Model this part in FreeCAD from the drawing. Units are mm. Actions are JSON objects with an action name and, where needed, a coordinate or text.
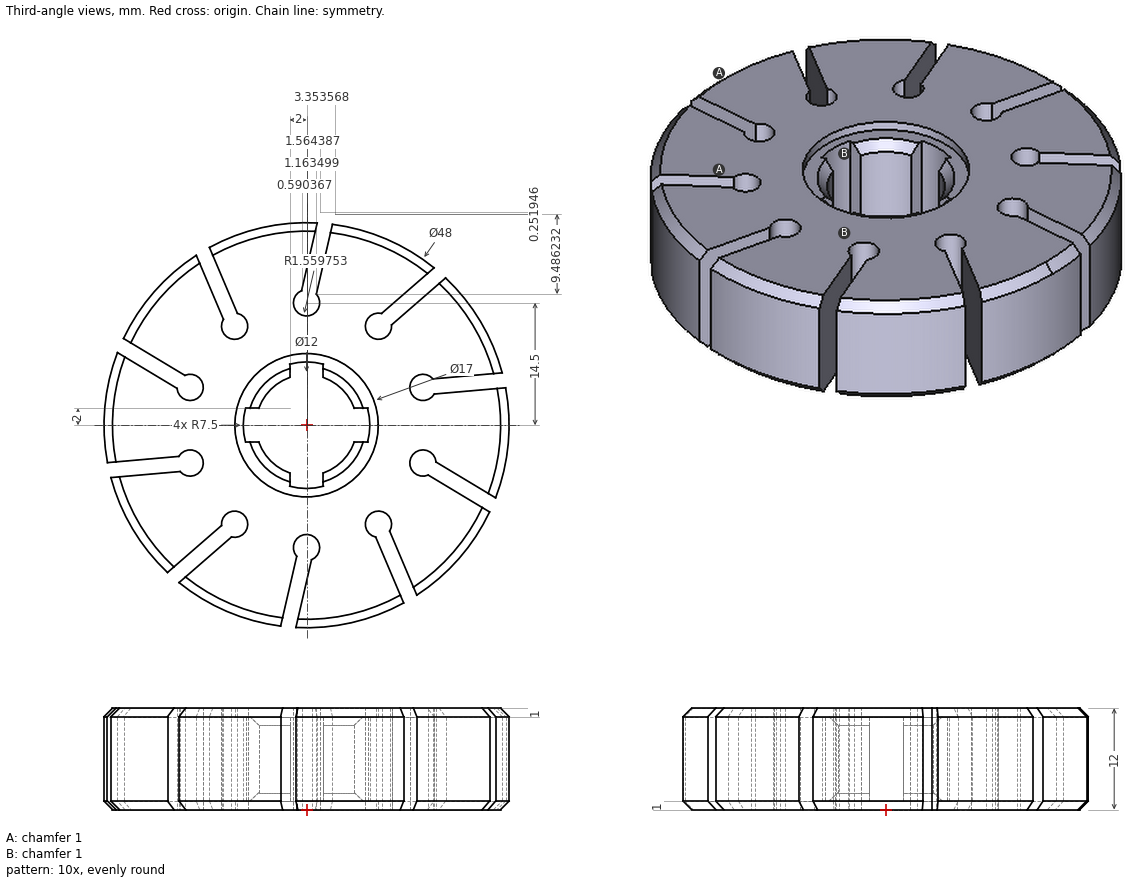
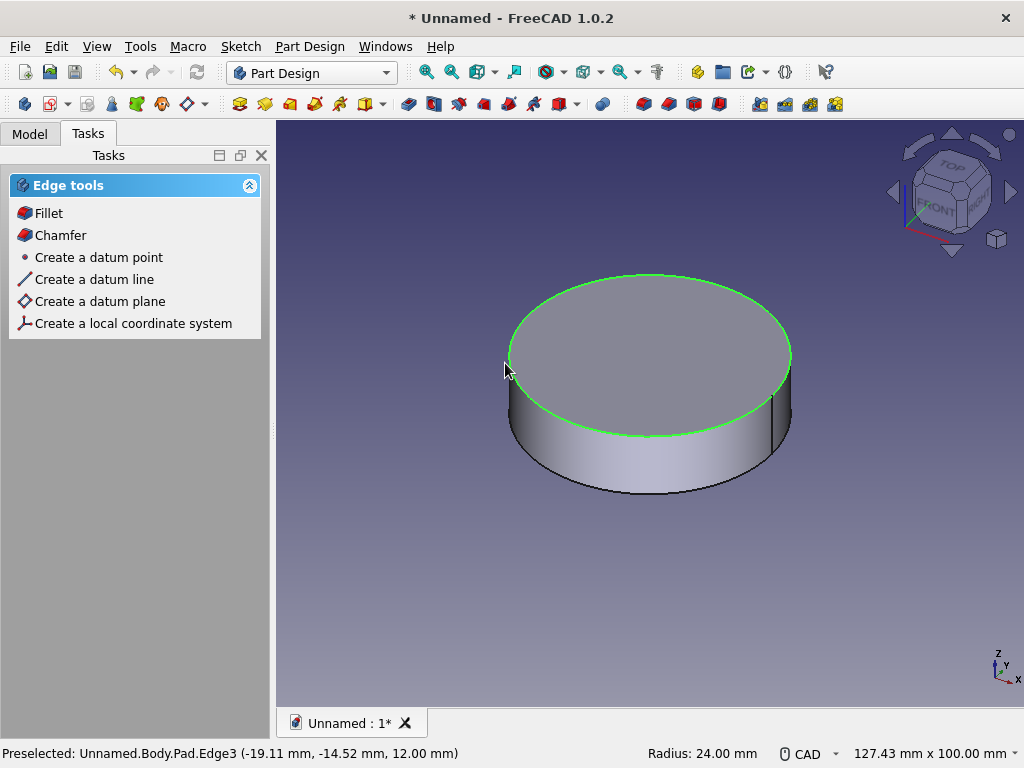
{"action": "key", "text": "0"}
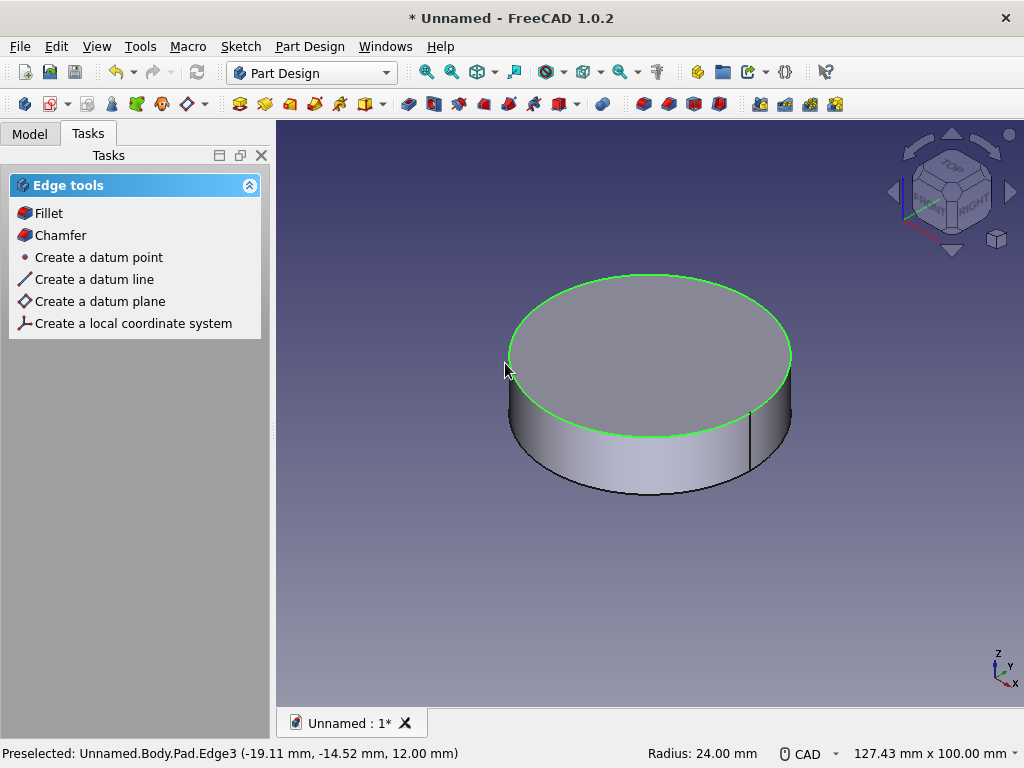
{"action": "key", "text": "2"}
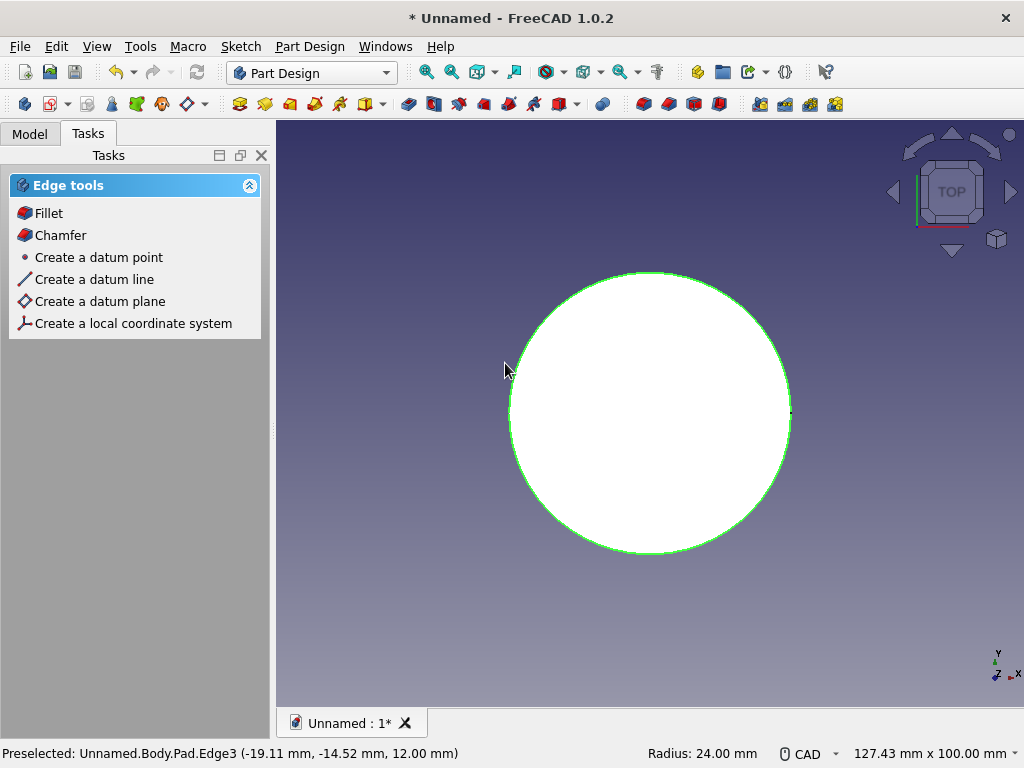
{"action": "key", "text": "1"}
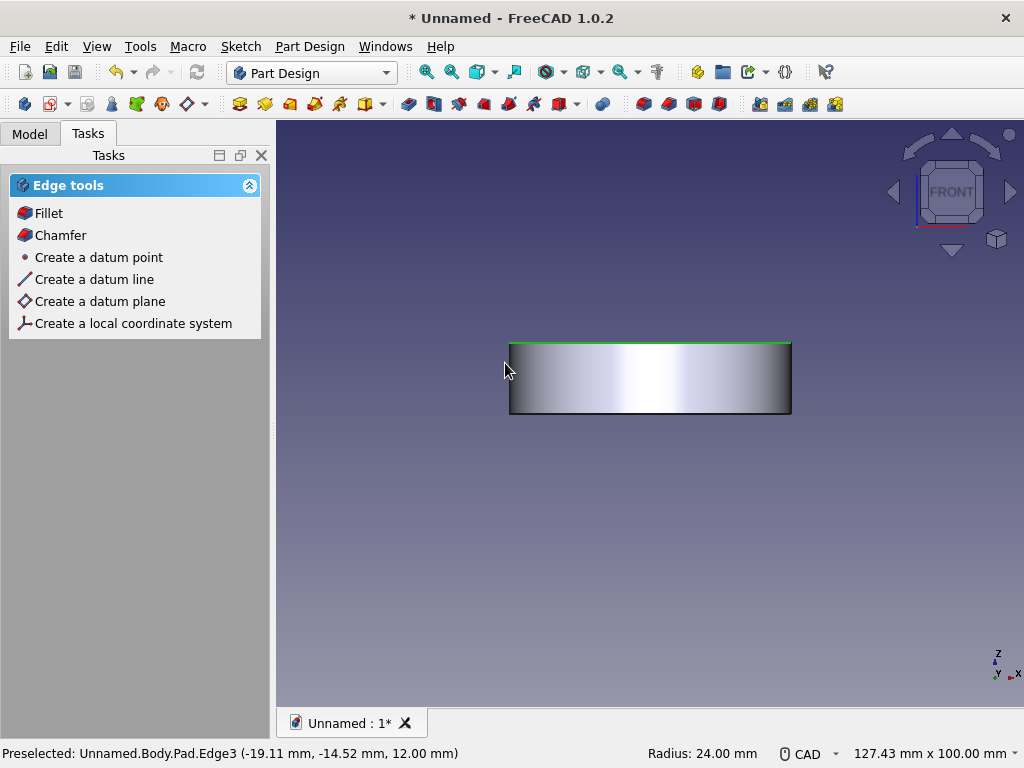
{"action": "left_click", "coordinate": [427, 72]}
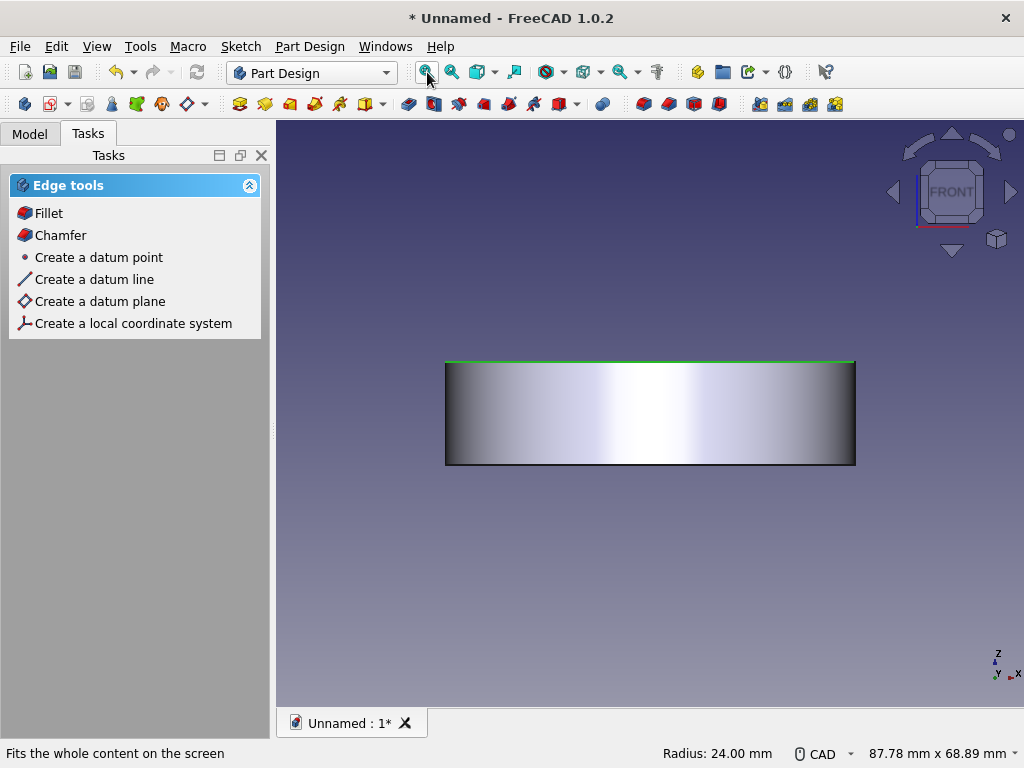
{"action": "left_click", "coordinate": [485, 464], "text": "ctrl"}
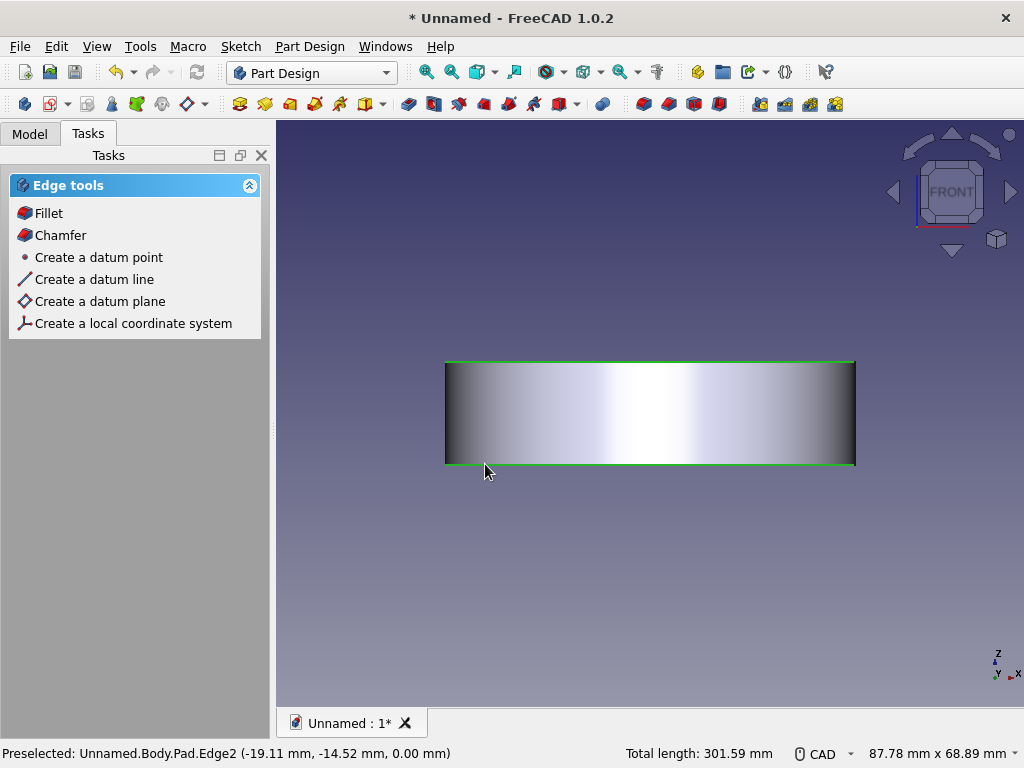
{"action": "left_click", "coordinate": [669, 104]}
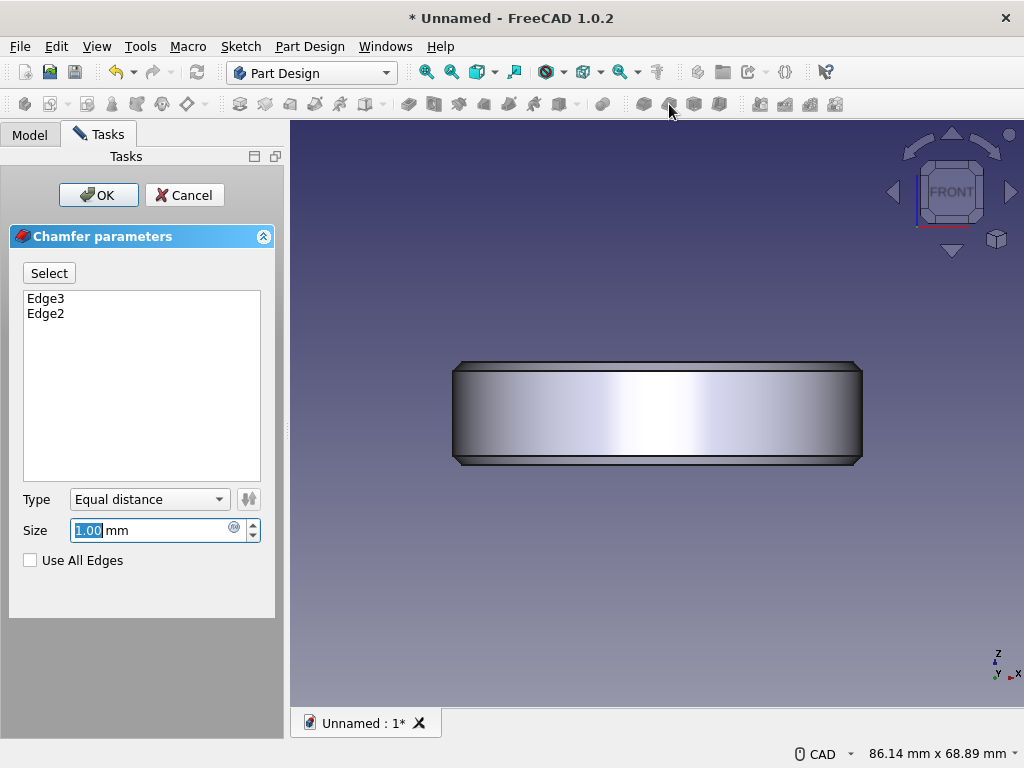
{"action": "type", "text": "1"}
{"action": "key", "text": "Tab"}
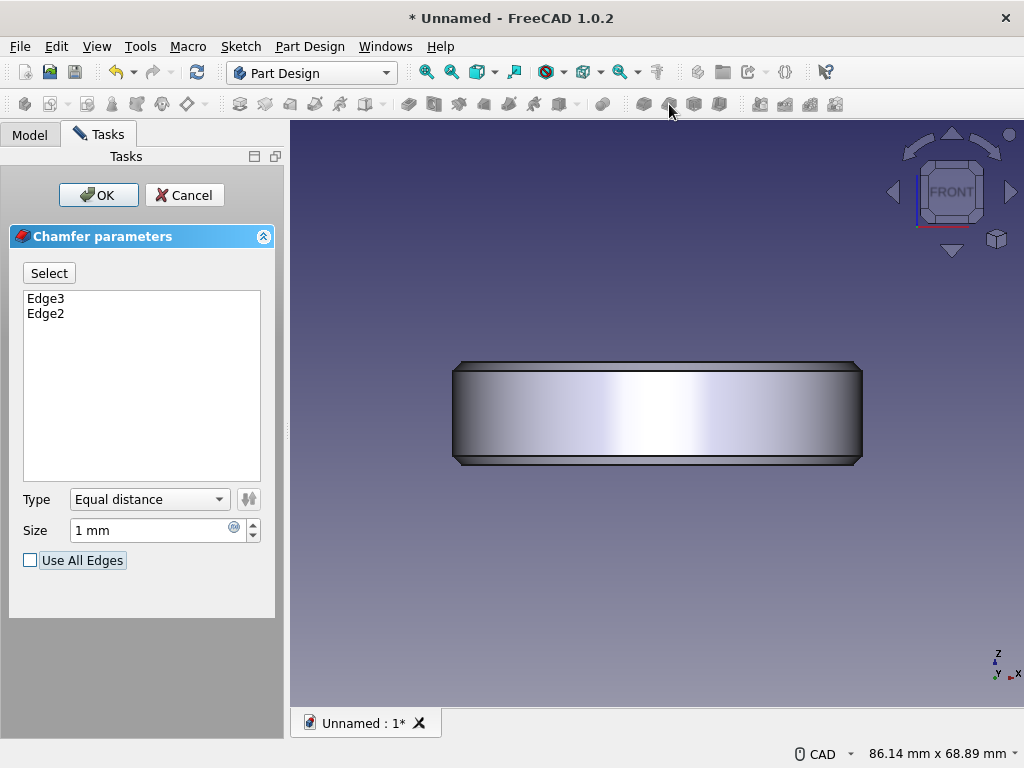
{"action": "left_click", "coordinate": [99, 195]}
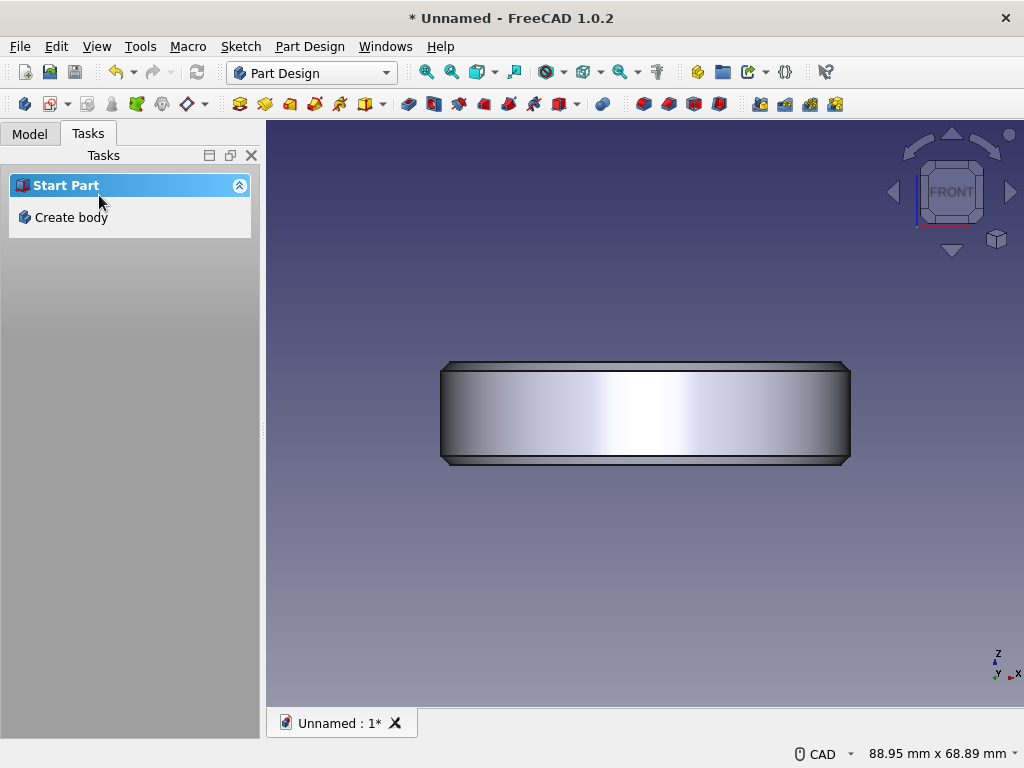
{"action": "key", "text": "0"}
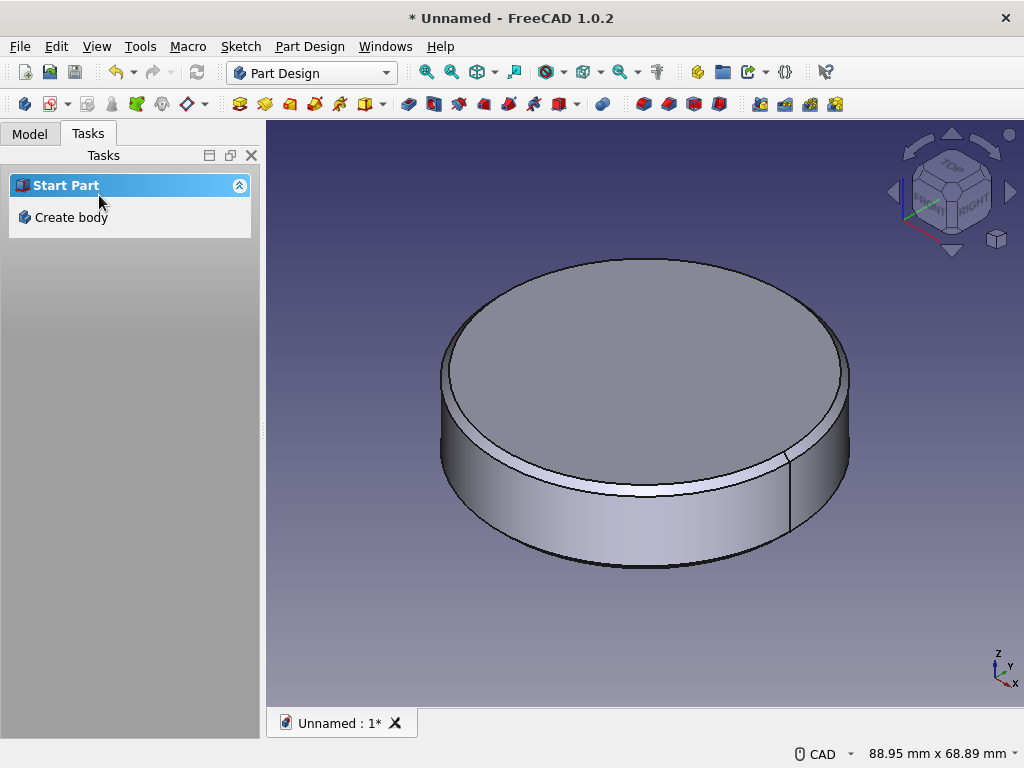
{"action": "left_click", "coordinate": [645, 371]}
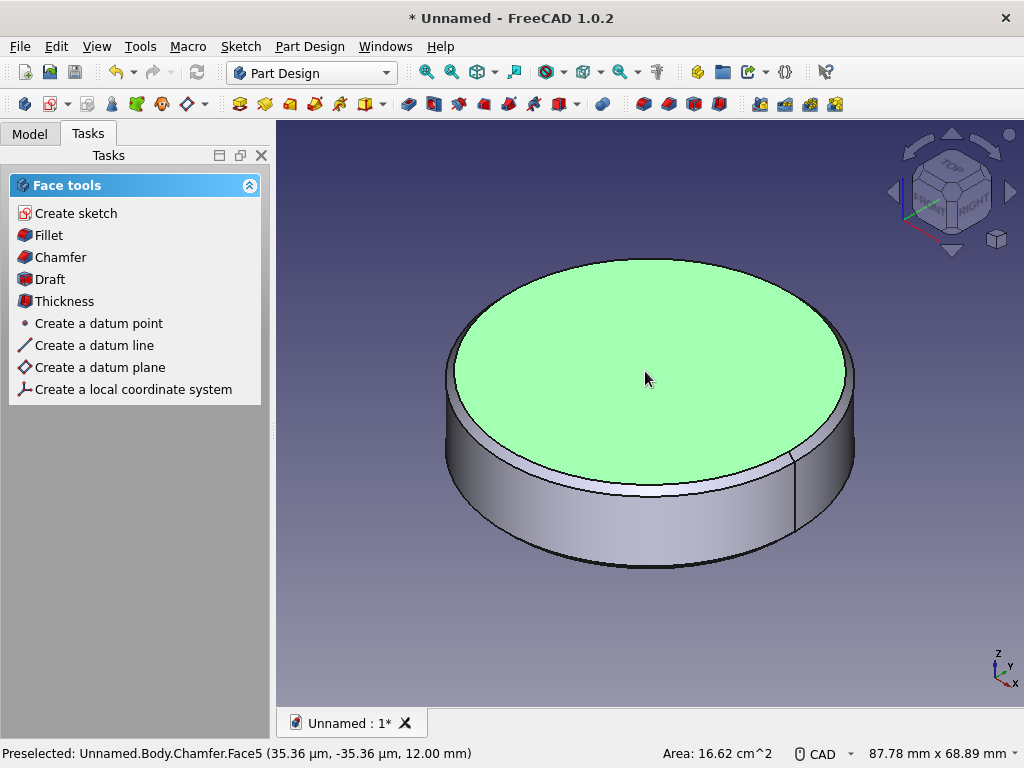
{"action": "left_click", "coordinate": [50, 104]}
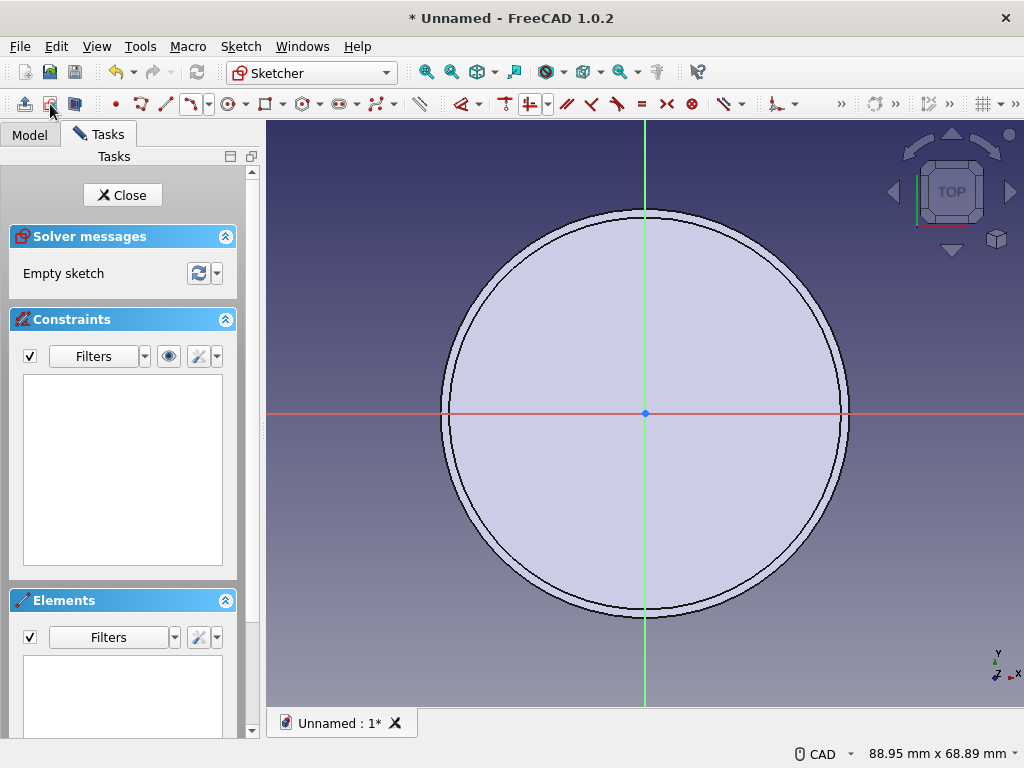
{"action": "scroll", "coordinate": [685, 414], "scroll_direction": "up", "scroll_amount": 5}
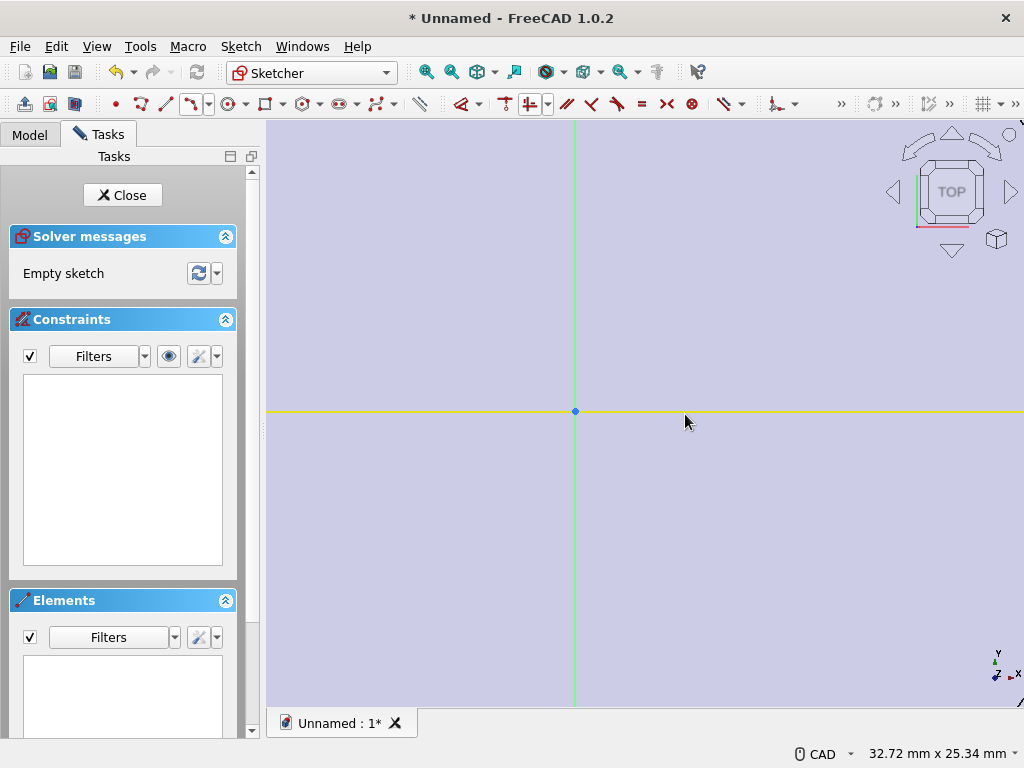
{"action": "left_click", "coordinate": [228, 104]}